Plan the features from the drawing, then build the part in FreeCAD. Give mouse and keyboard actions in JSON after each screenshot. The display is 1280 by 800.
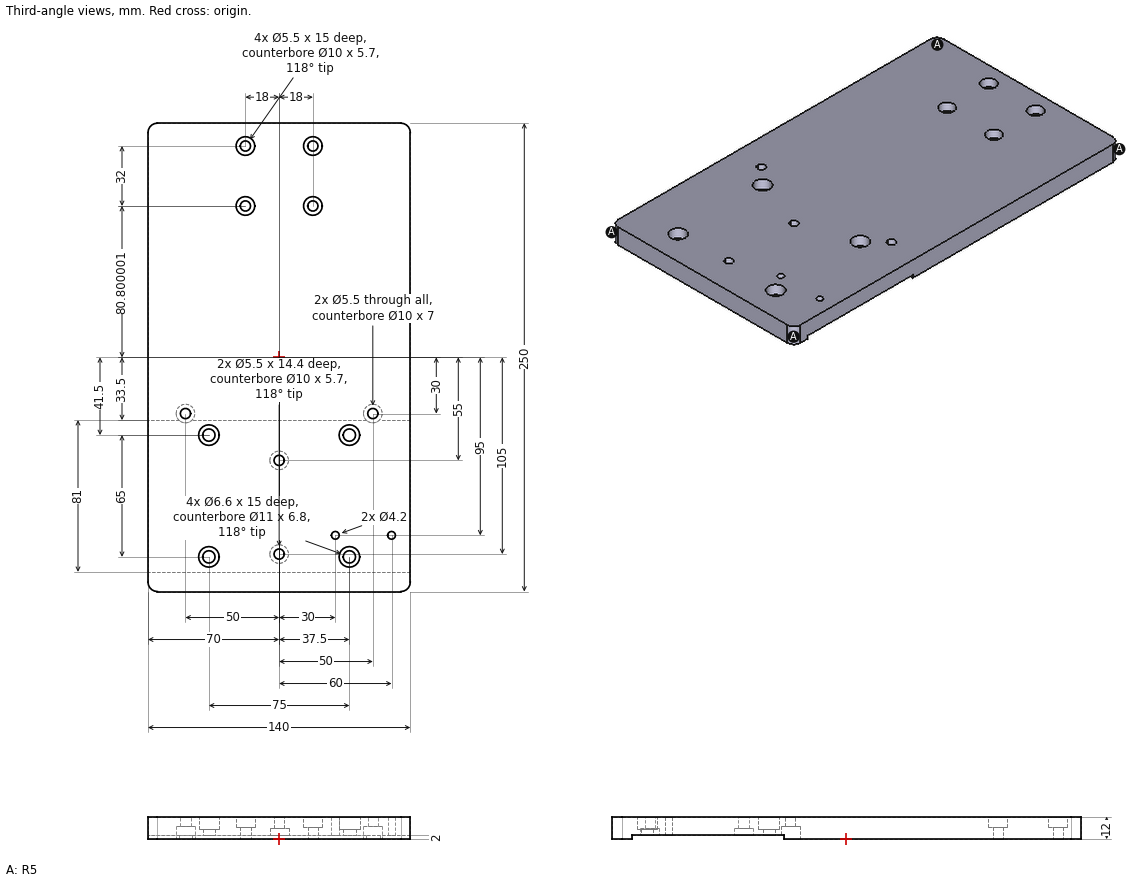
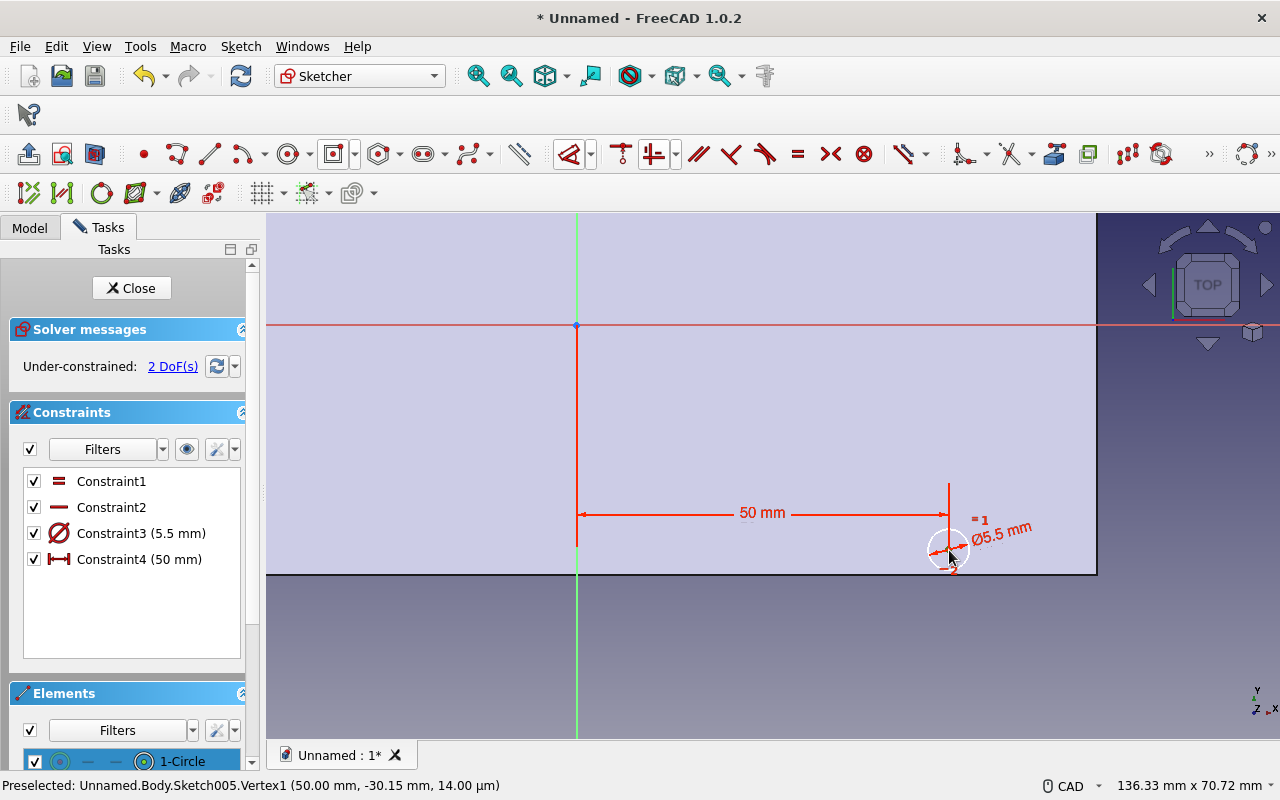
{"action": "left_click", "coordinate": [590, 154]}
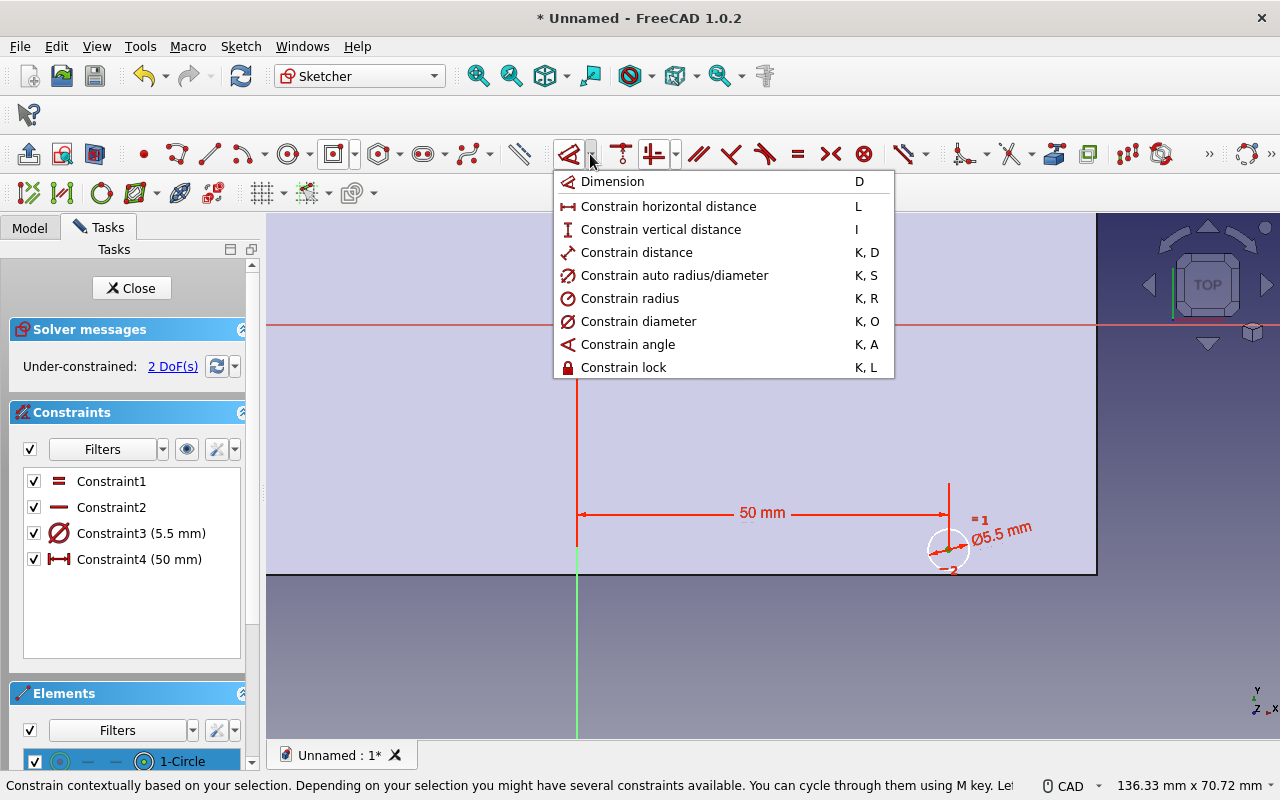
{"action": "left_click", "coordinate": [724, 230]}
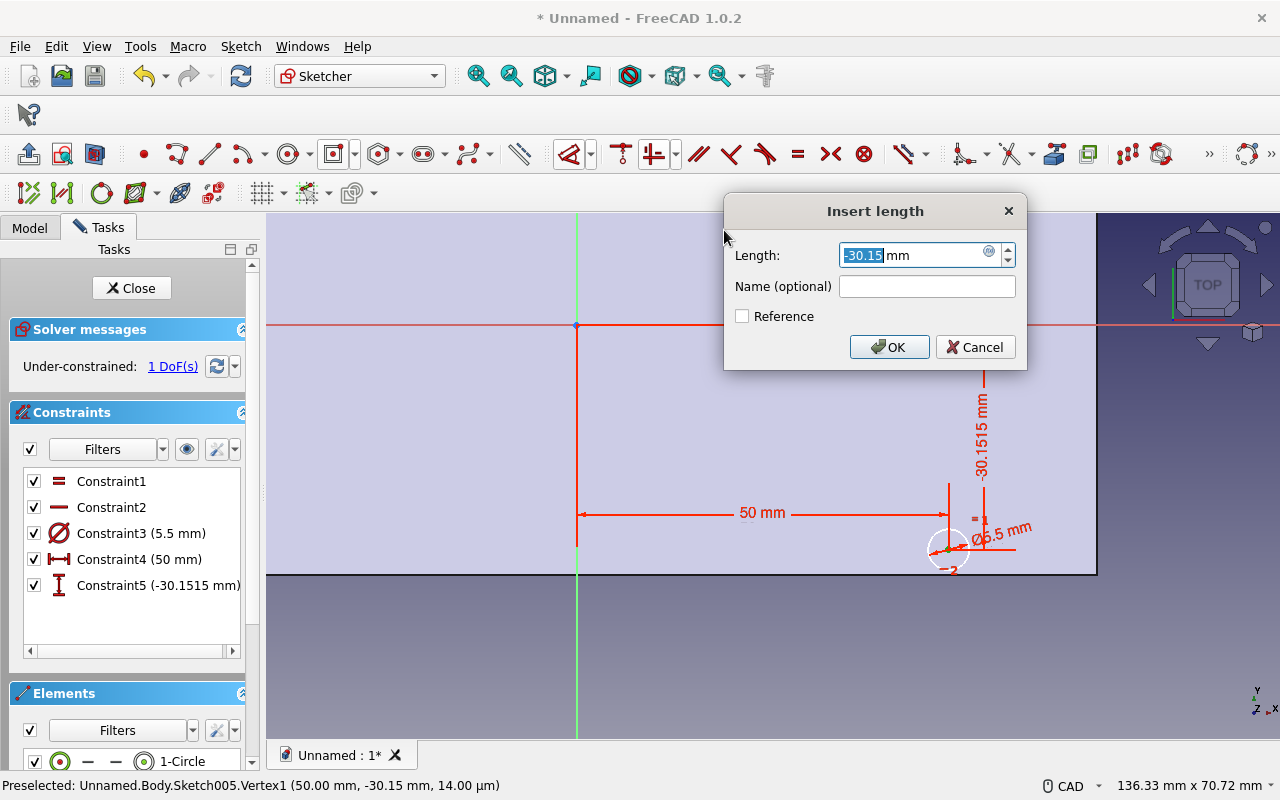
{"action": "type", "text": "-30"}
{"action": "key", "text": "Return"}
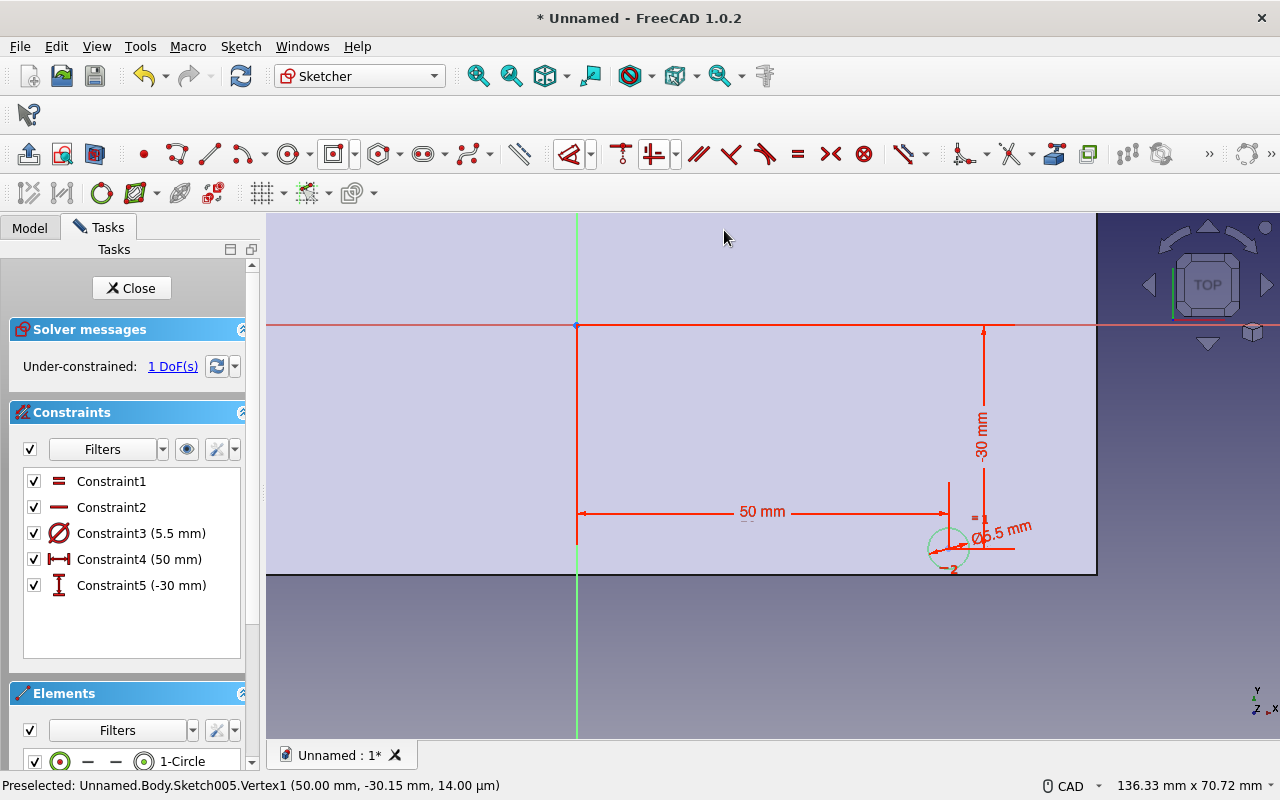
{"action": "scroll", "coordinate": [964, 534], "scroll_direction": "down", "scroll_amount": 2}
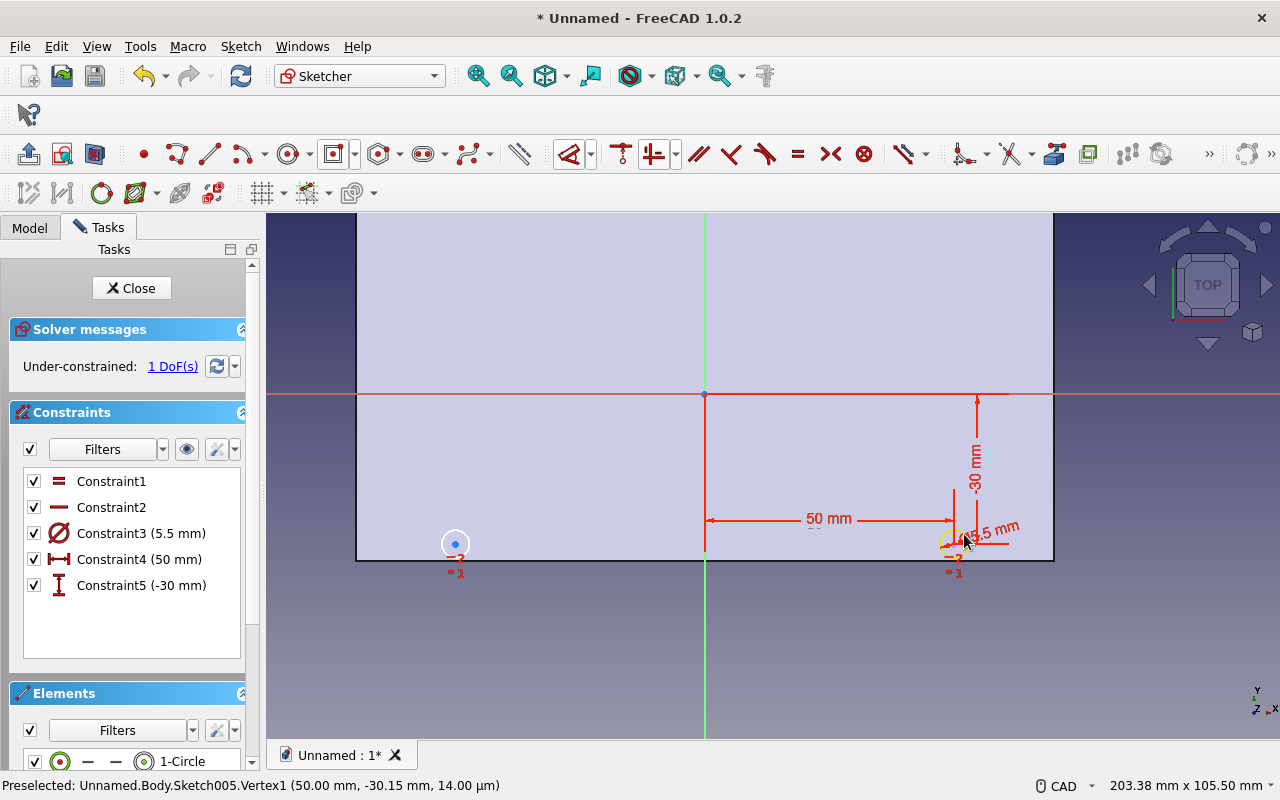
{"action": "left_click", "coordinate": [456, 544]}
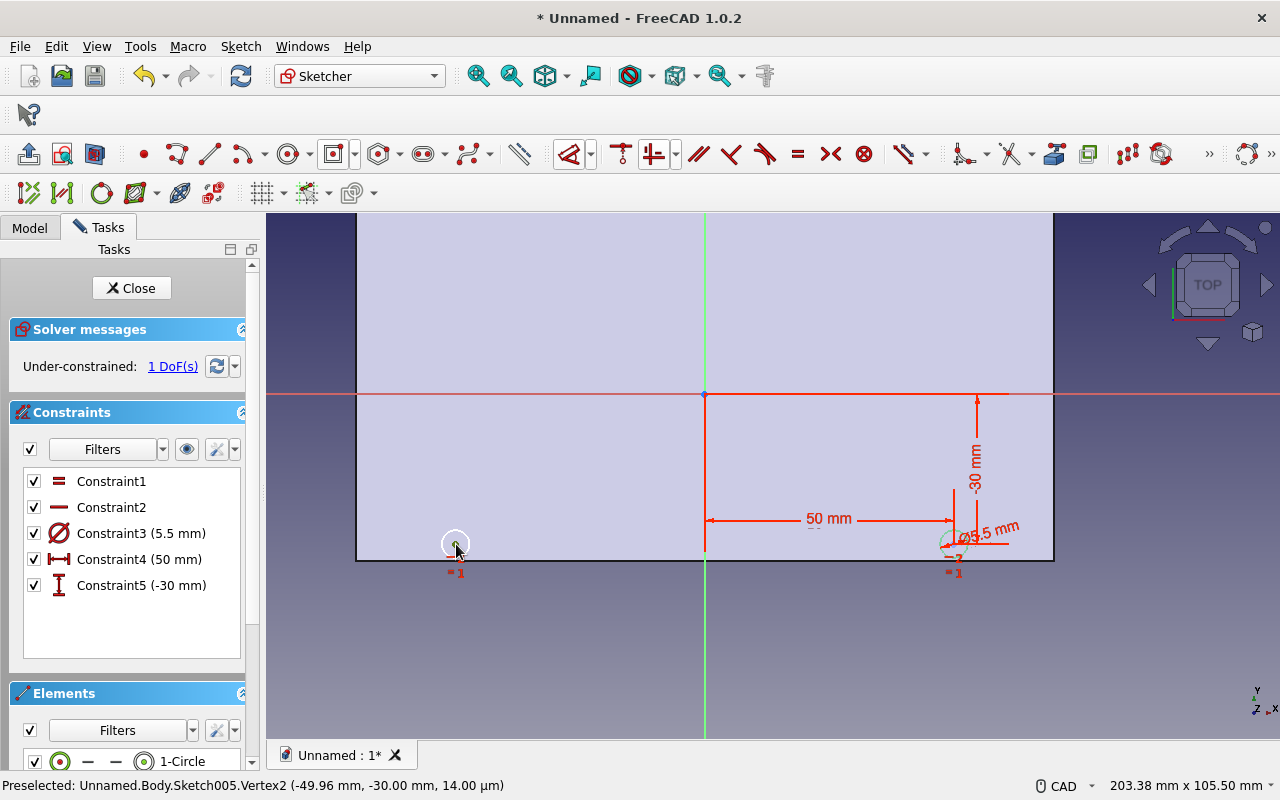
{"action": "left_click", "coordinate": [590, 154]}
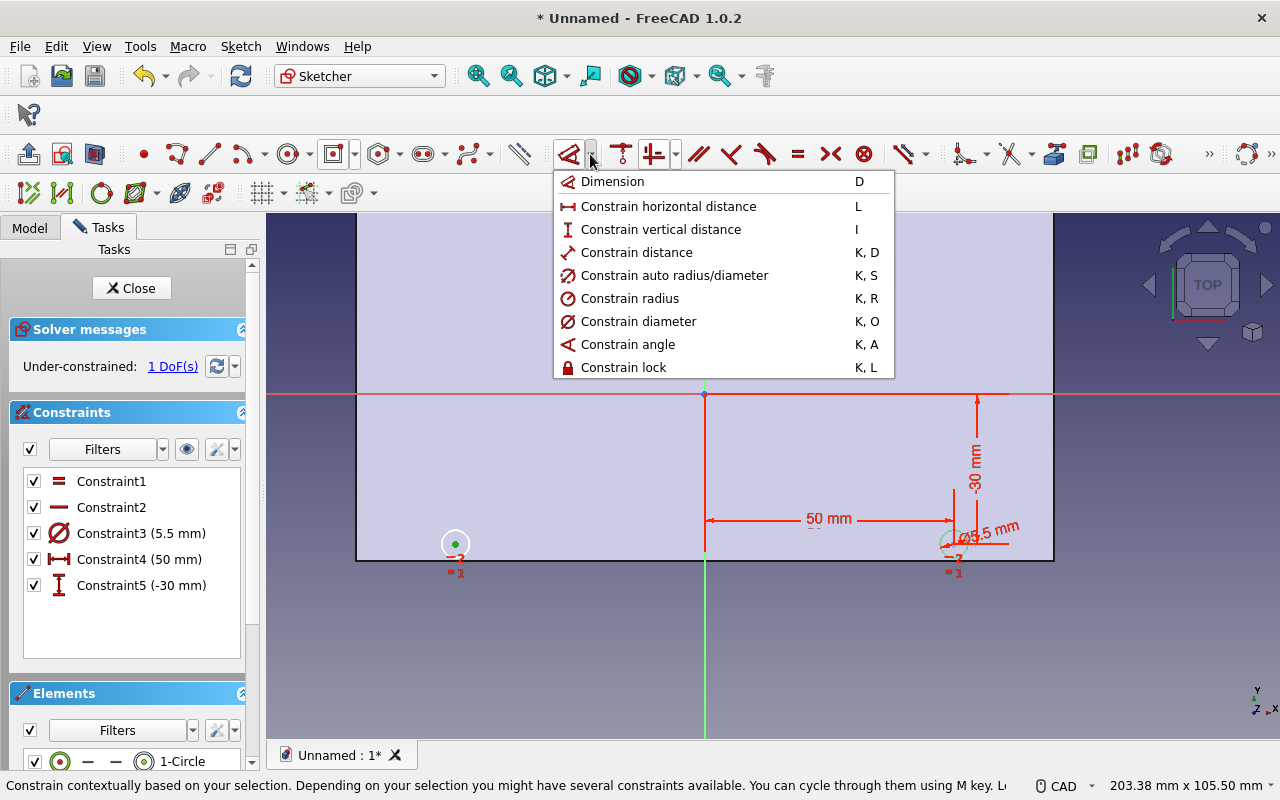
{"action": "left_click", "coordinate": [724, 206]}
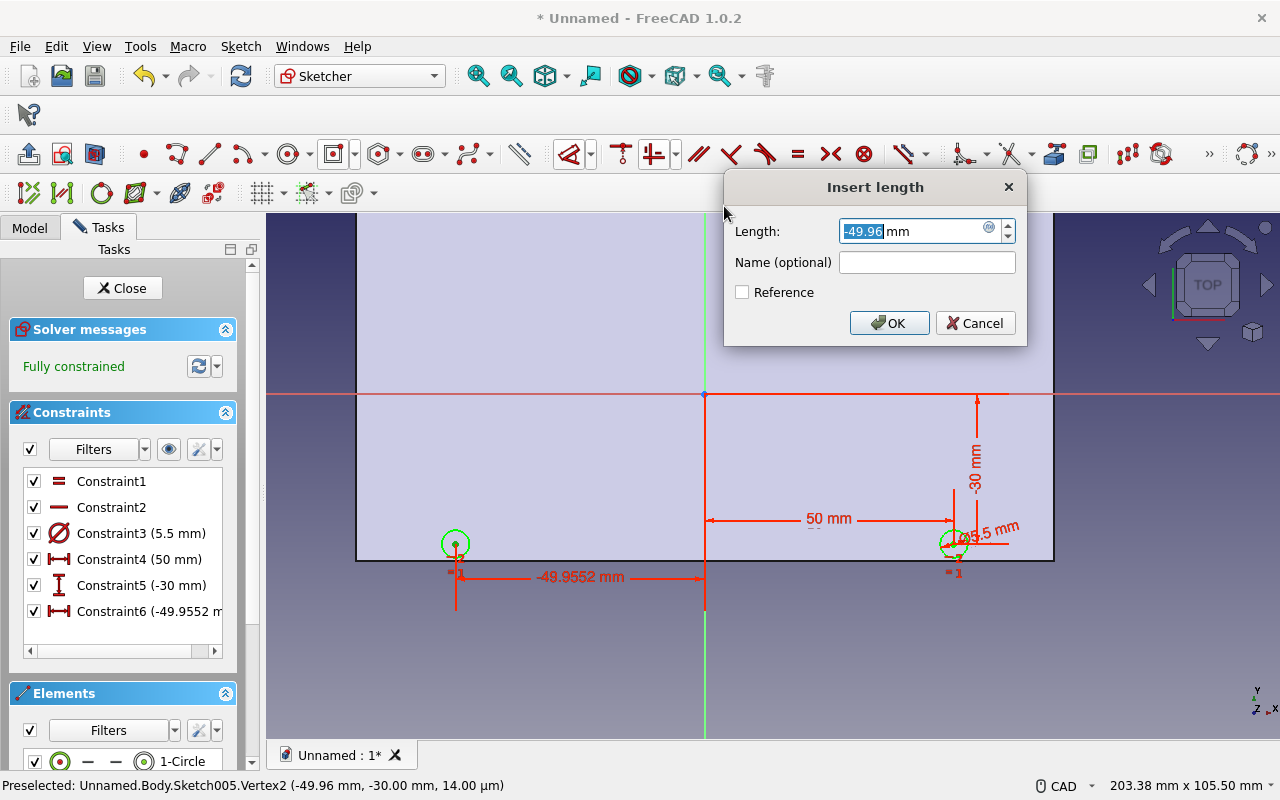
{"action": "type", "text": "-50"}
{"action": "key", "text": "Return"}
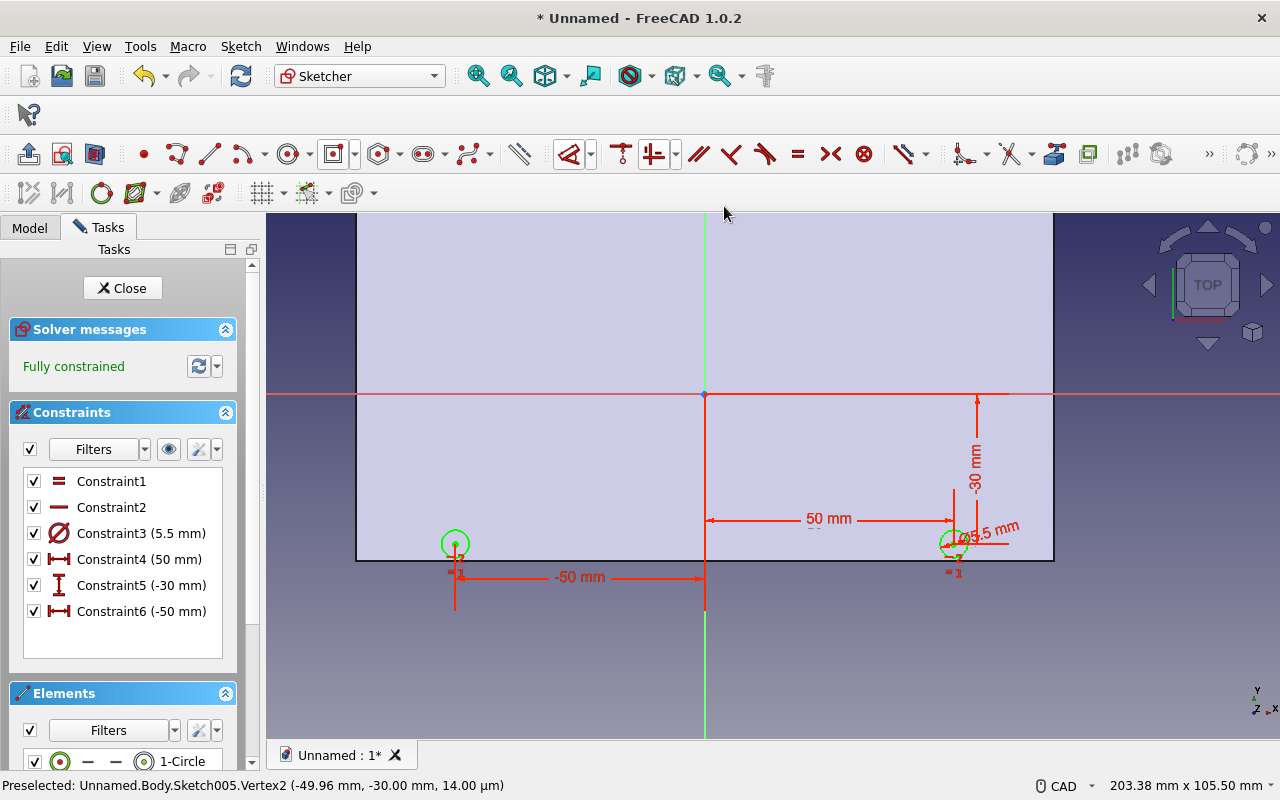
{"action": "left_click", "coordinate": [123, 288]}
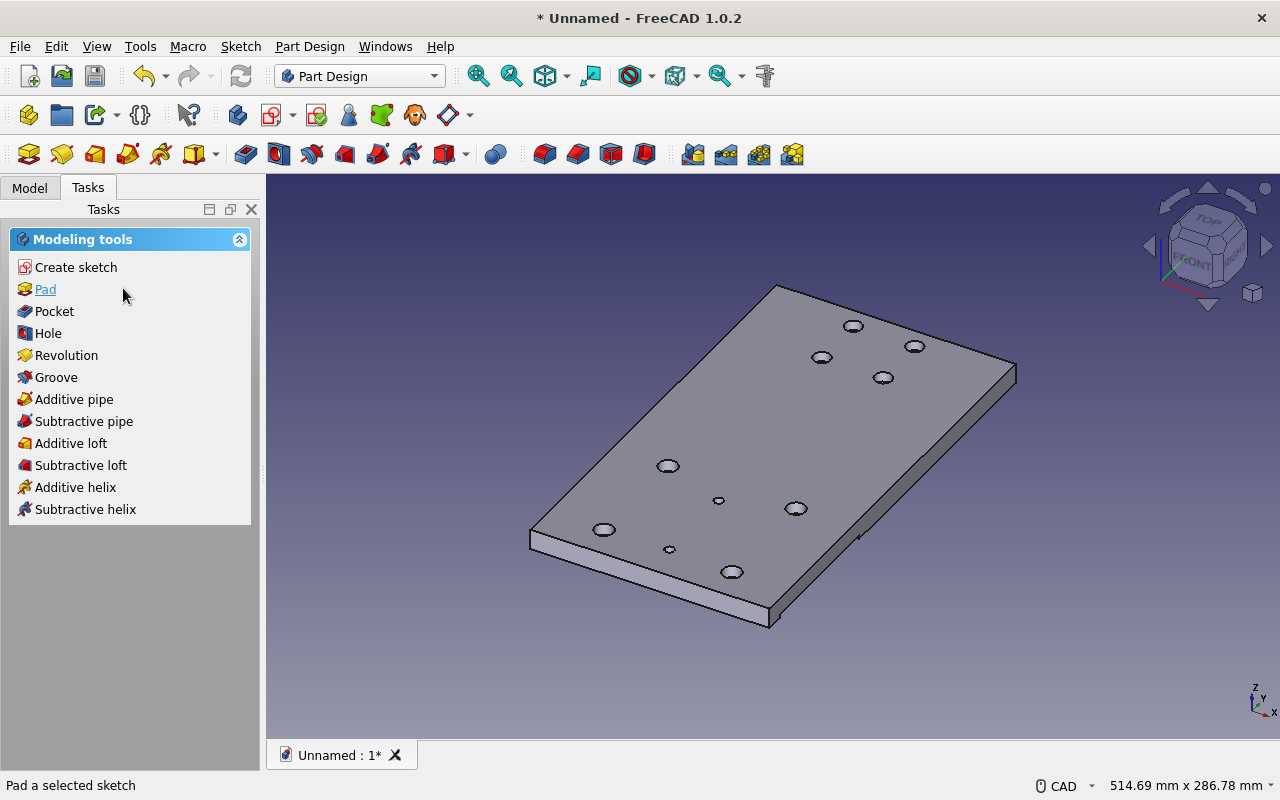
{"action": "left_click", "coordinate": [279, 154]}